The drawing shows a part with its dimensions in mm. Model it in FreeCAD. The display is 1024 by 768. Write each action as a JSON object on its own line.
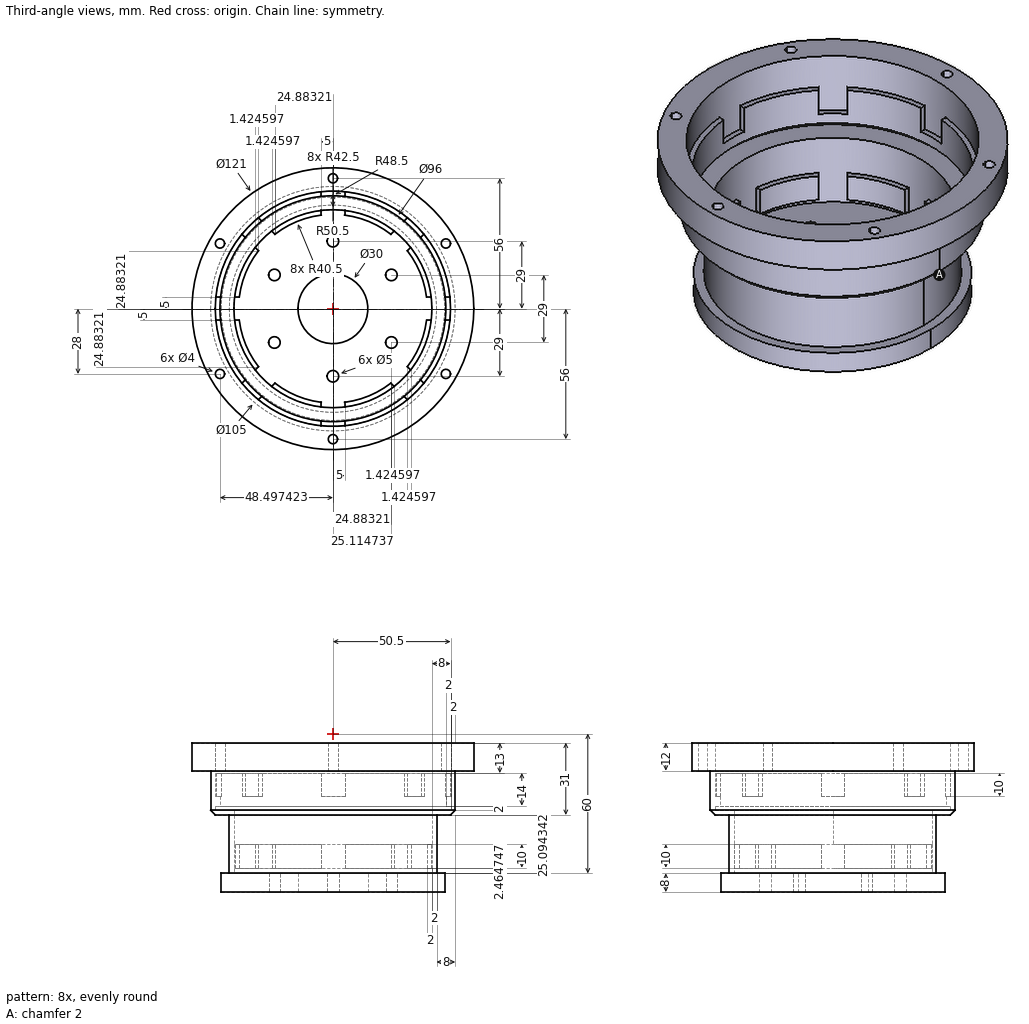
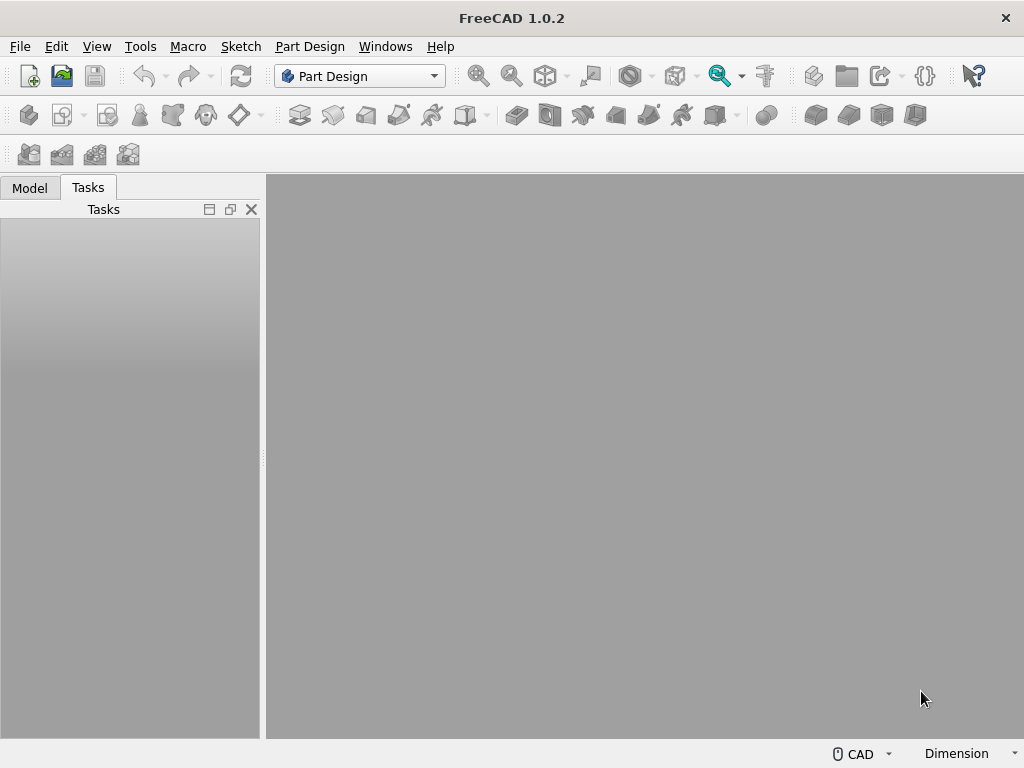
{"action": "left_click", "coordinate": [29, 76]}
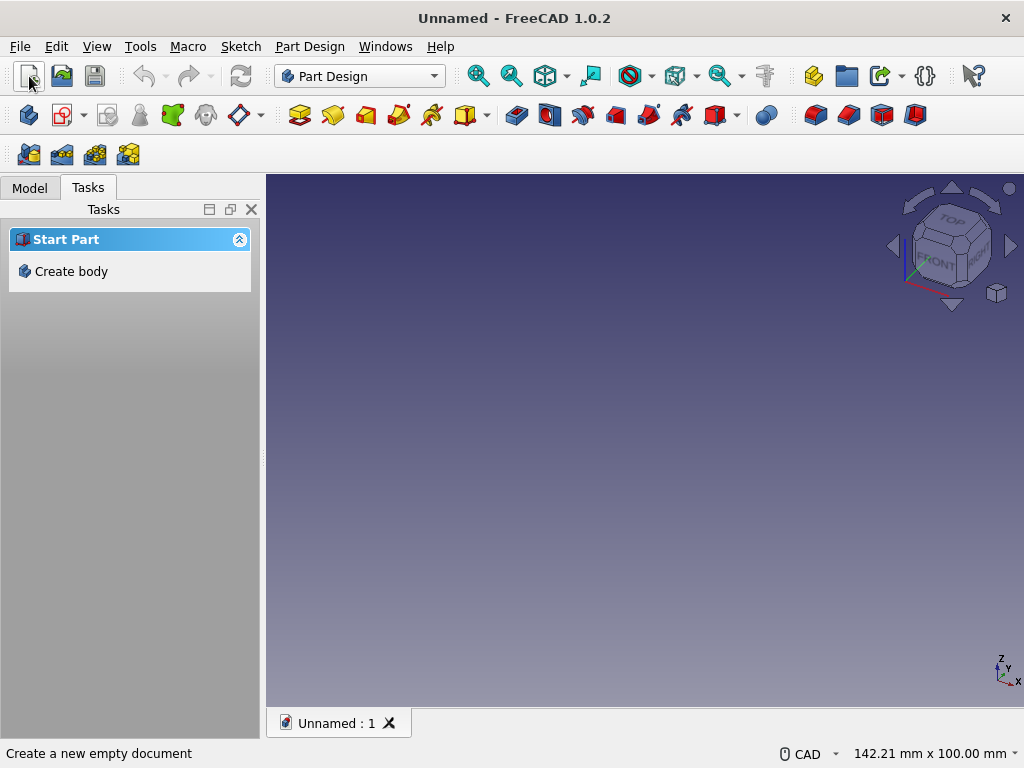
{"action": "left_click", "coordinate": [62, 116]}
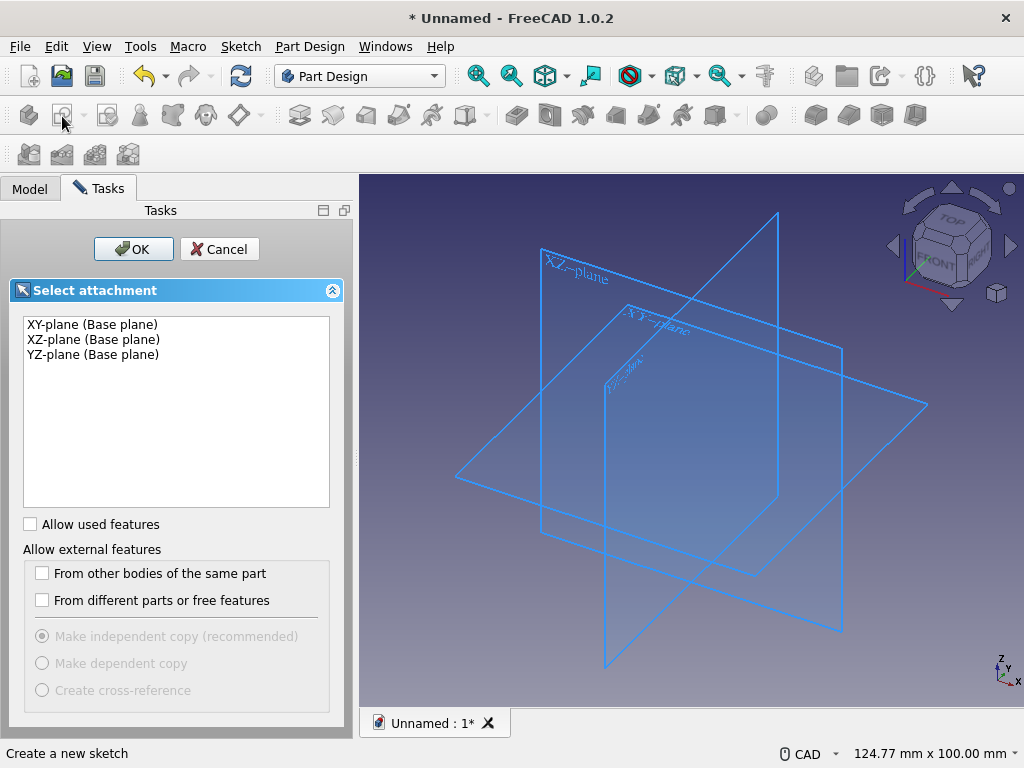
{"action": "left_click", "coordinate": [84, 340]}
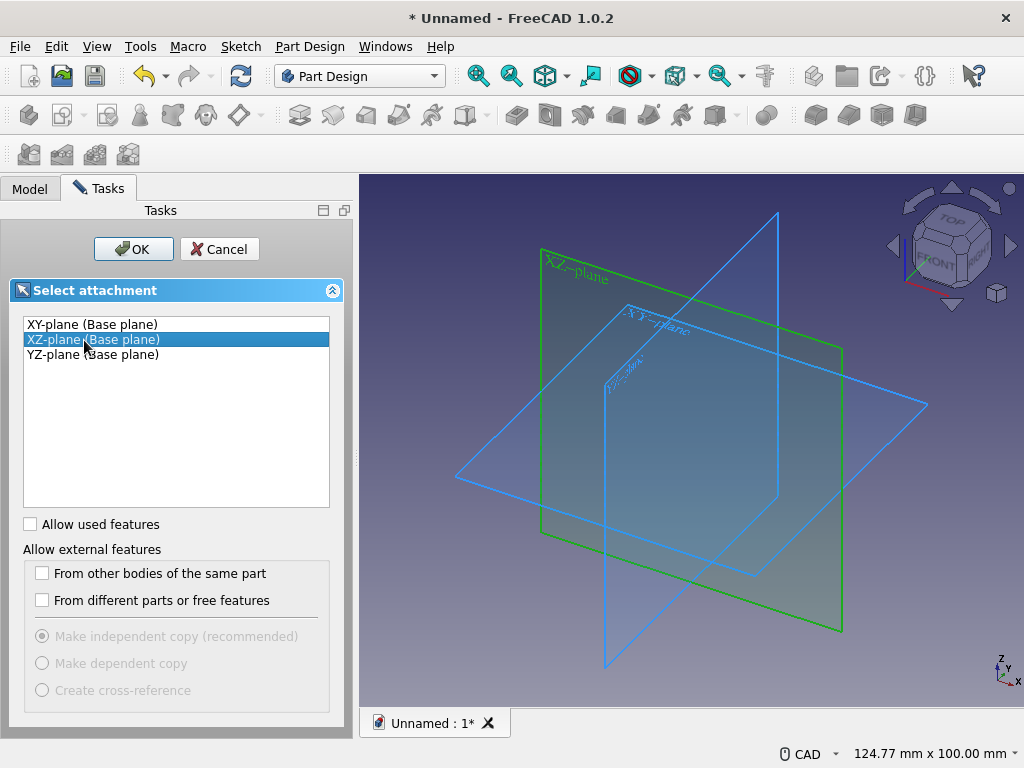
{"action": "left_click", "coordinate": [134, 249]}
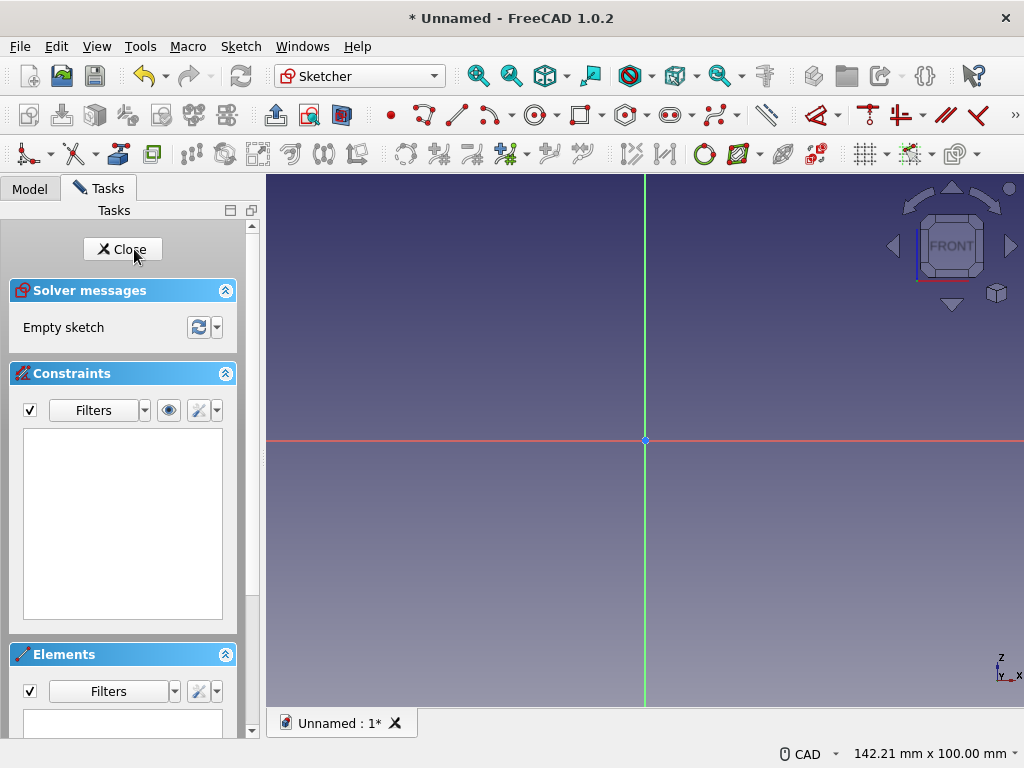
{"action": "scroll", "coordinate": [294, 202], "scroll_direction": "down", "scroll_amount": 2}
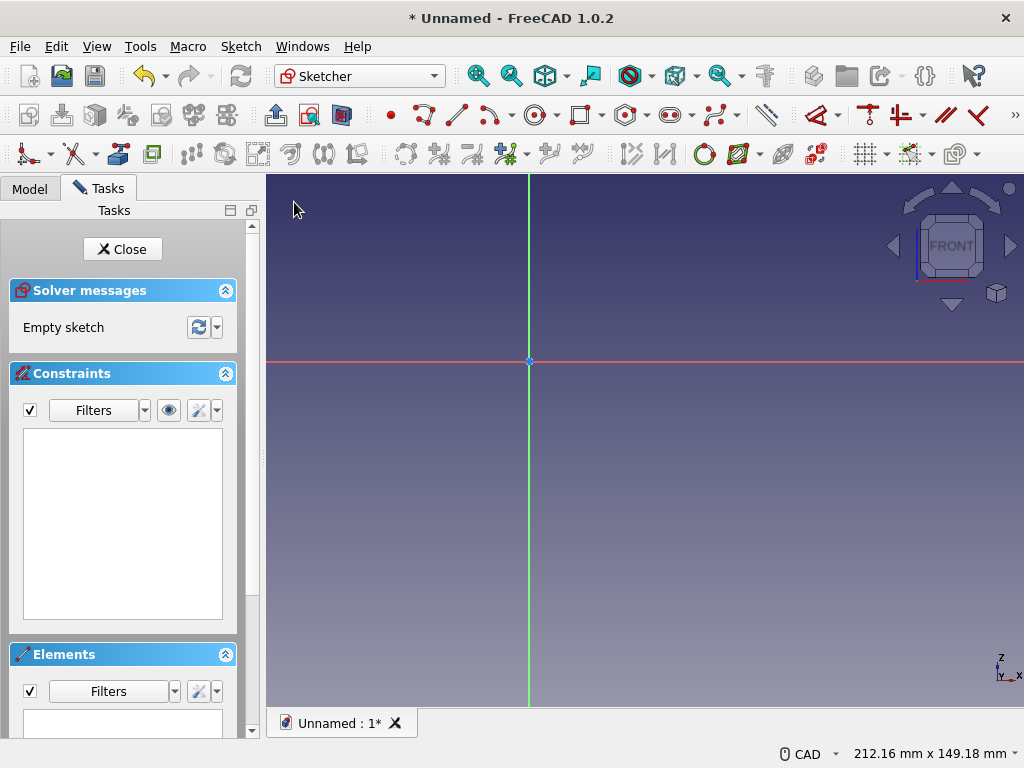
{"action": "scroll", "coordinate": [718, 527], "scroll_direction": "up", "scroll_amount": 2}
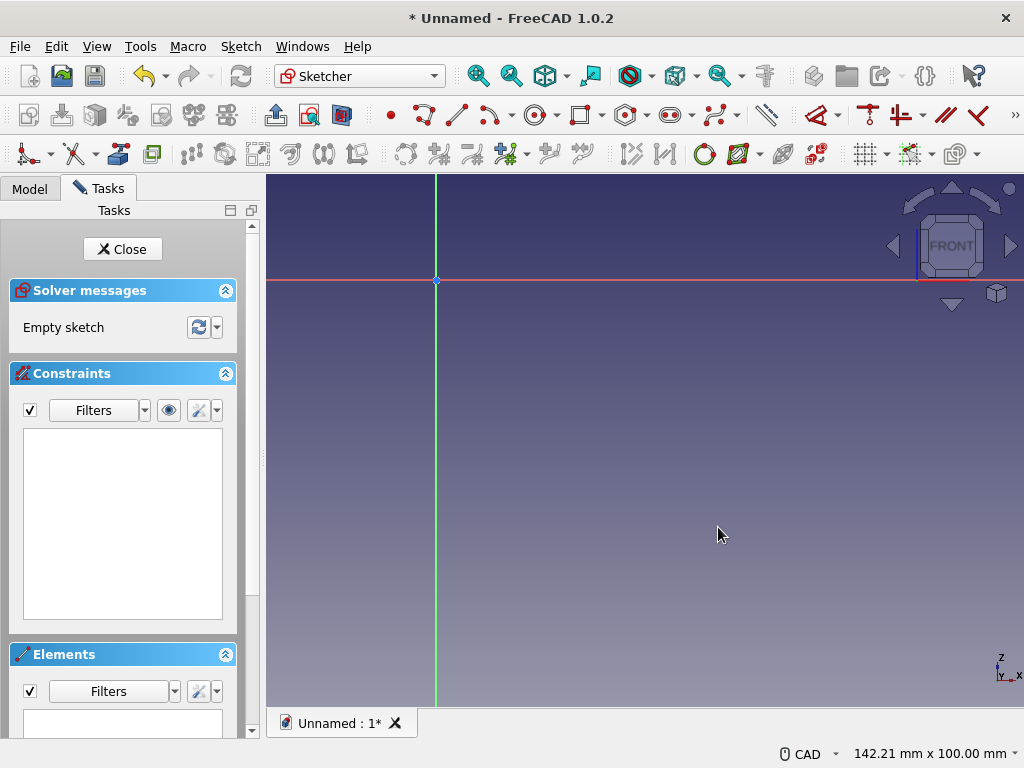
{"action": "key", "text": "g m"}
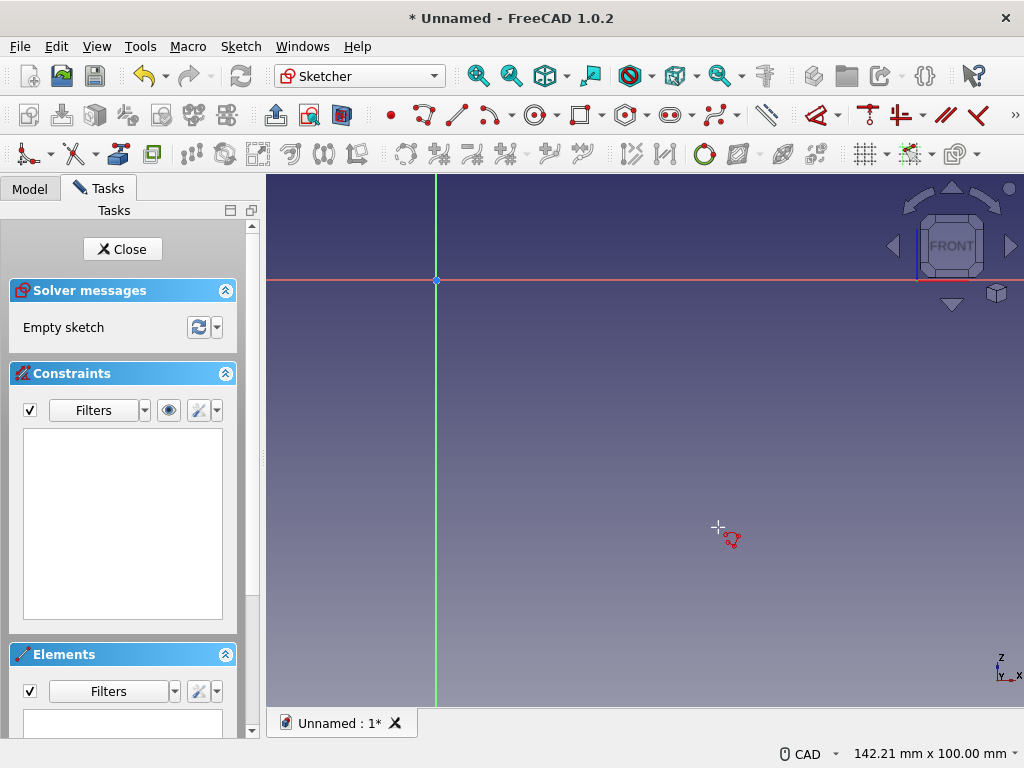
{"action": "left_click", "coordinate": [705, 301]}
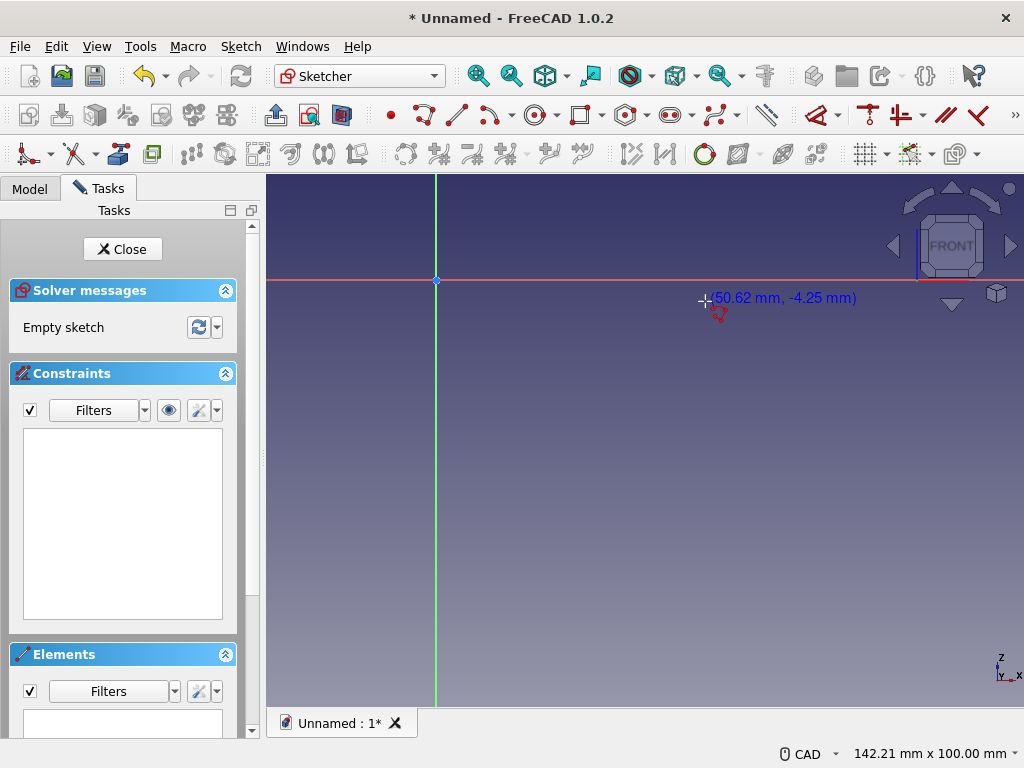
{"action": "scroll", "coordinate": [716, 301], "scroll_direction": "up", "scroll_amount": 2}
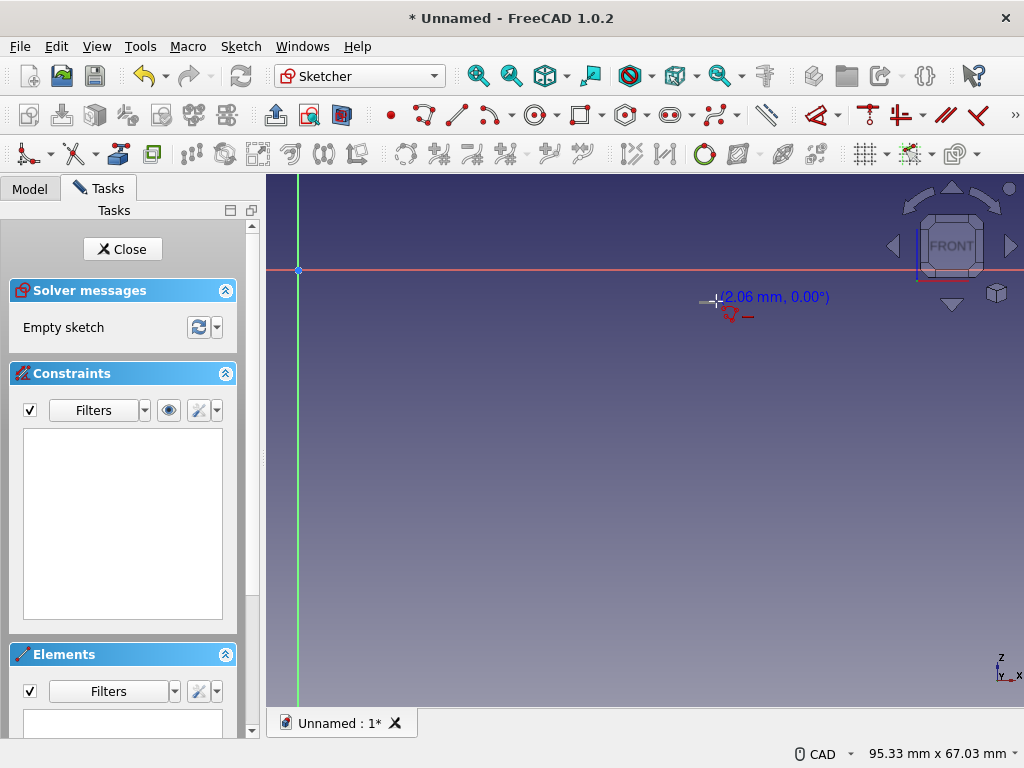
{"action": "left_click", "coordinate": [716, 301]}
{"action": "left_click", "coordinate": [716, 548]}
{"action": "left_click", "coordinate": [652, 548]}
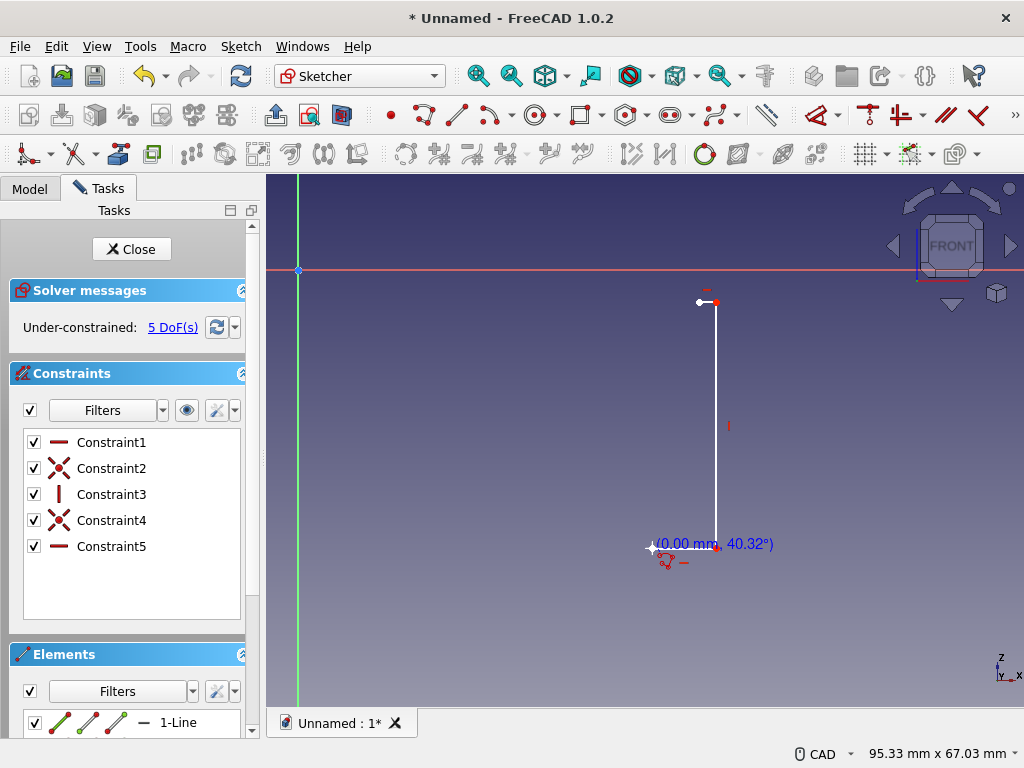
{"action": "scroll", "coordinate": [718, 302], "scroll_direction": "down", "scroll_amount": 2}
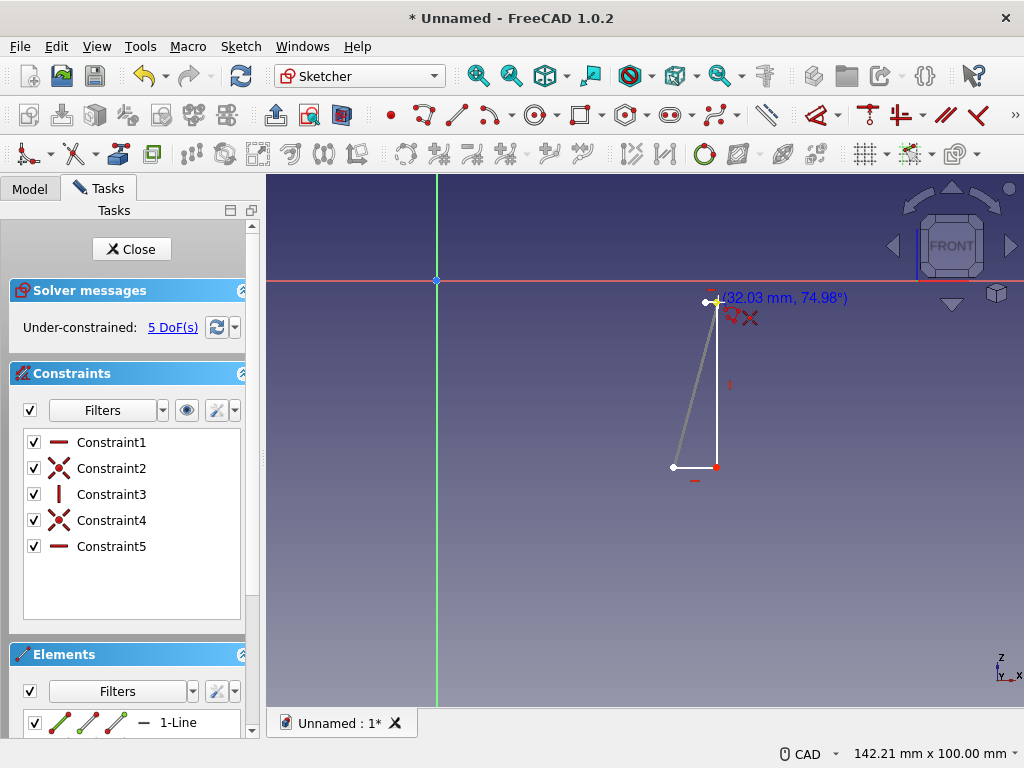
{"action": "left_click", "coordinate": [674, 600]}